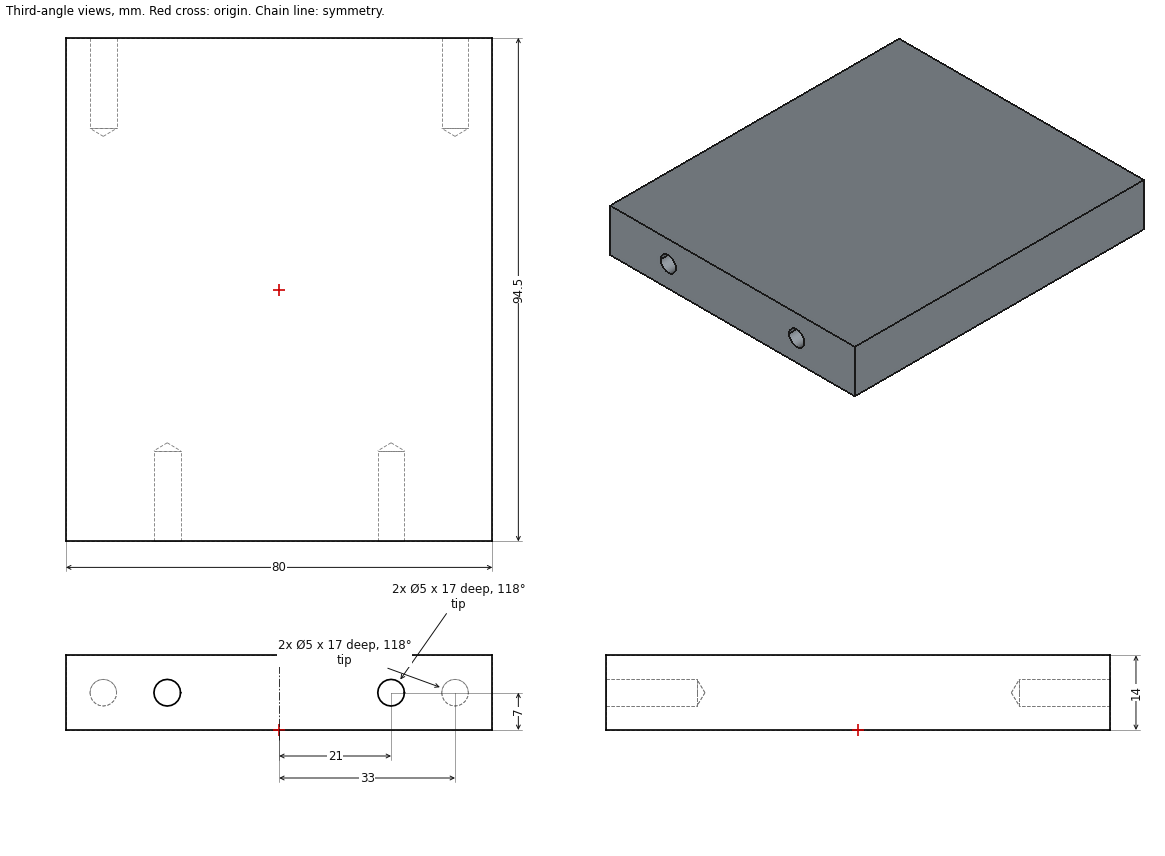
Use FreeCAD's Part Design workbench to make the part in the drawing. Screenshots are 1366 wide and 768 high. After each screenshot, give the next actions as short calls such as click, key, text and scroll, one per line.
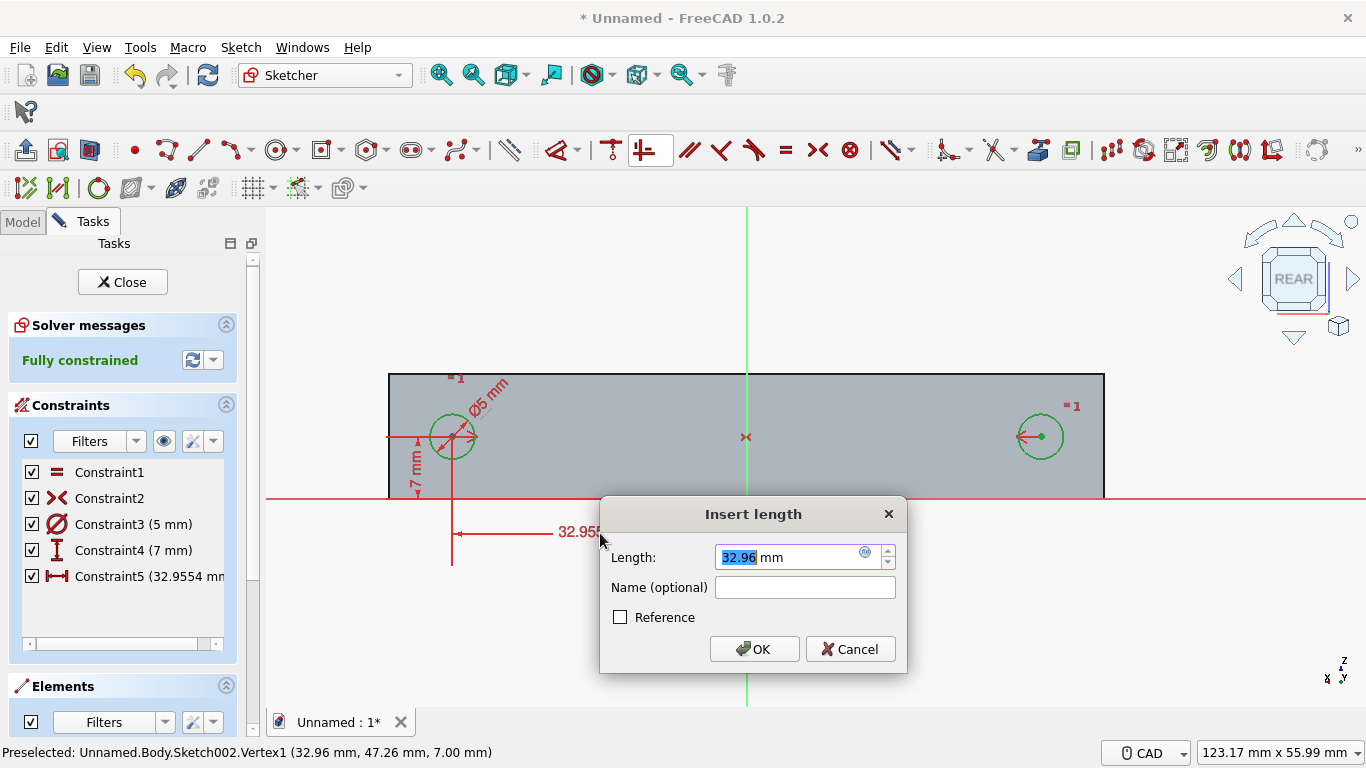
text(33)
key(Return)
key(Escape)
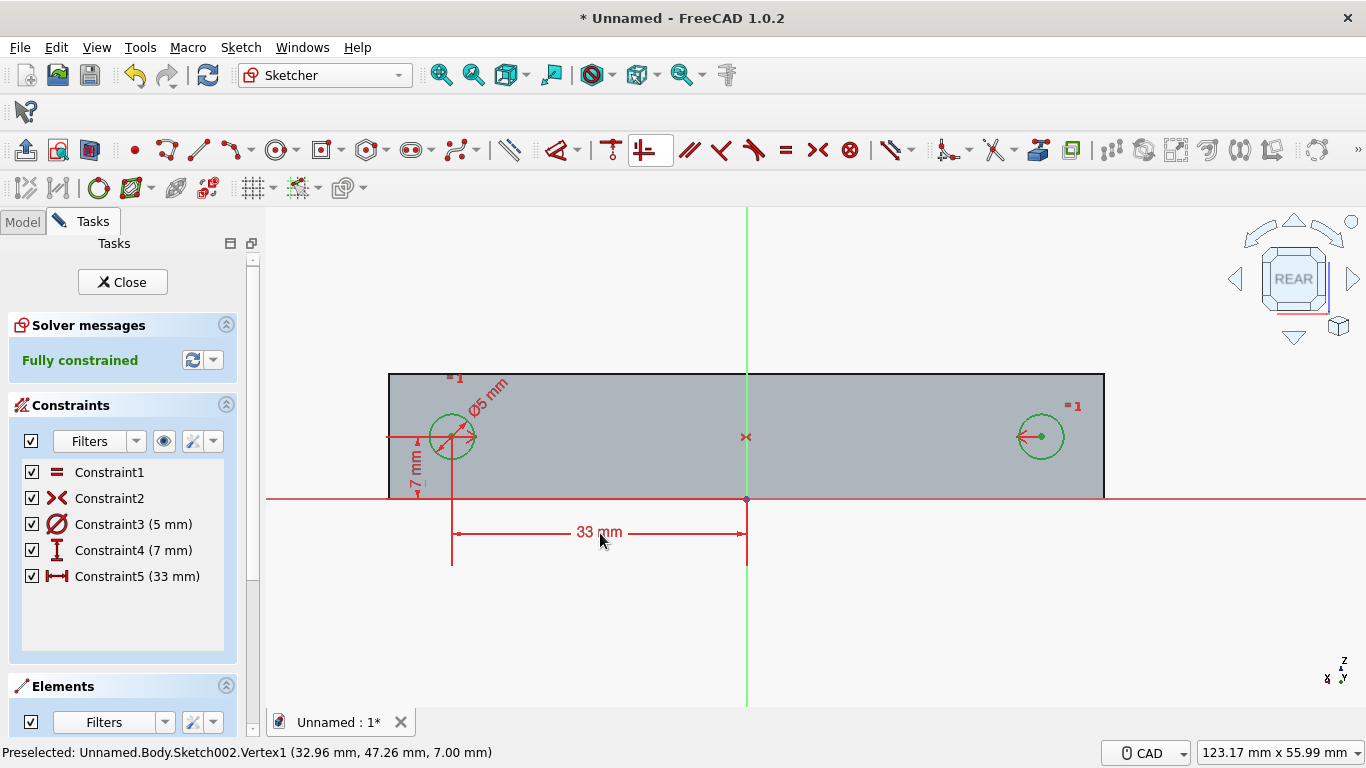
click(123, 282)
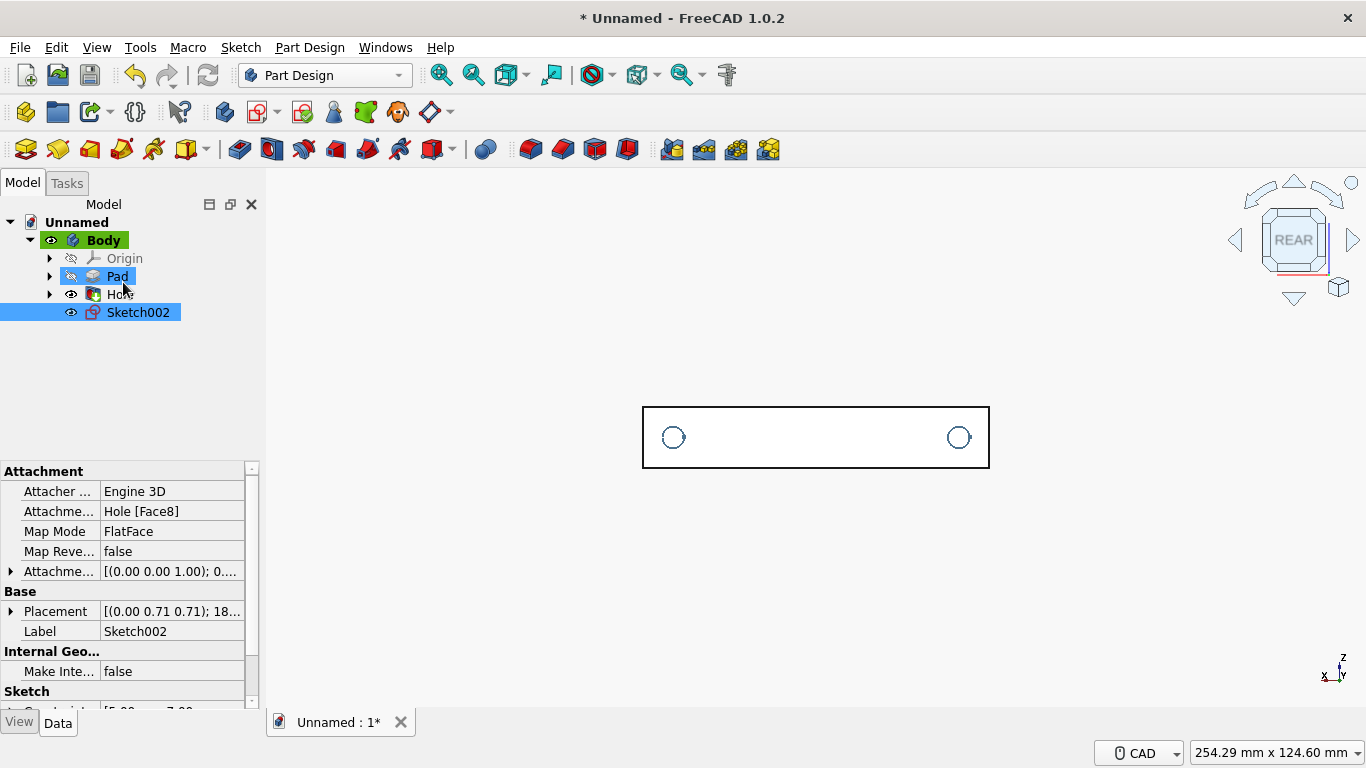
click(272, 150)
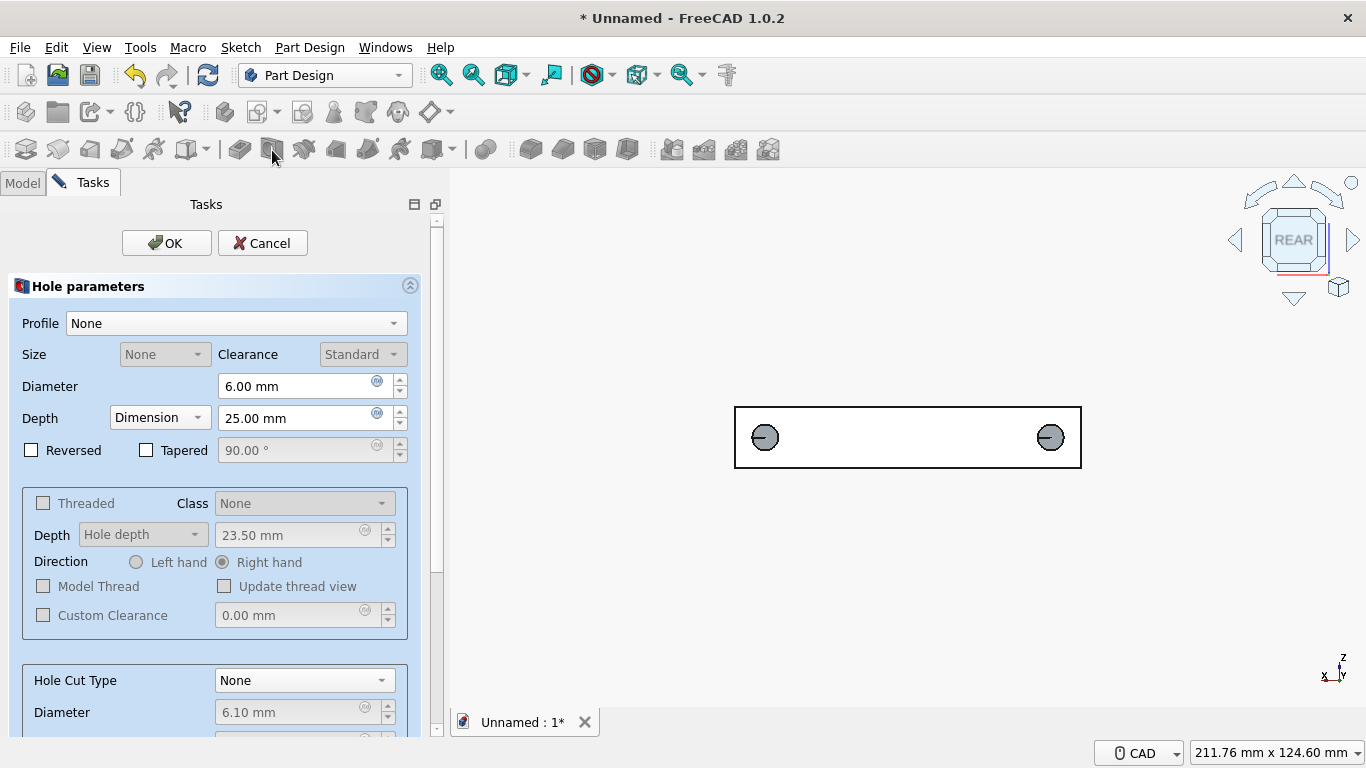
triple_click(305, 386)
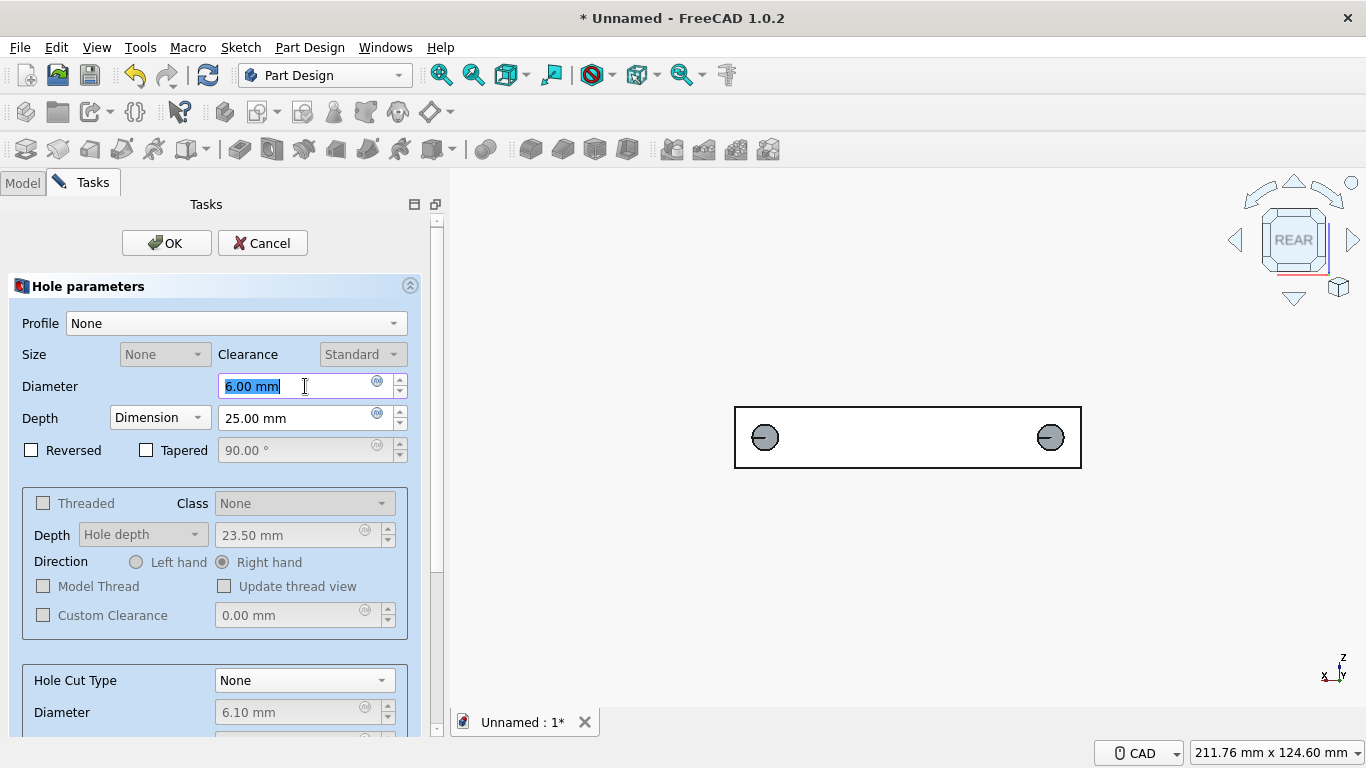
text(5)
key(Tab)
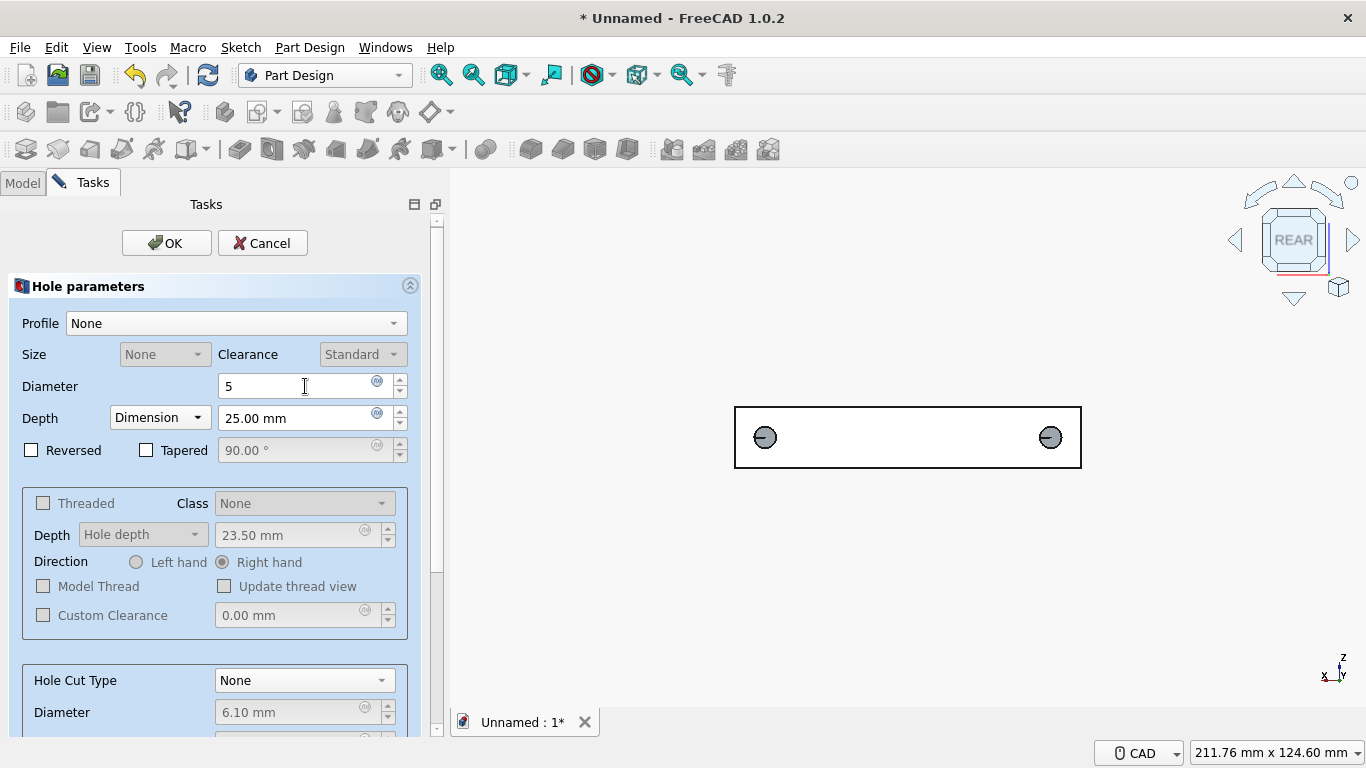
triple_click(305, 418)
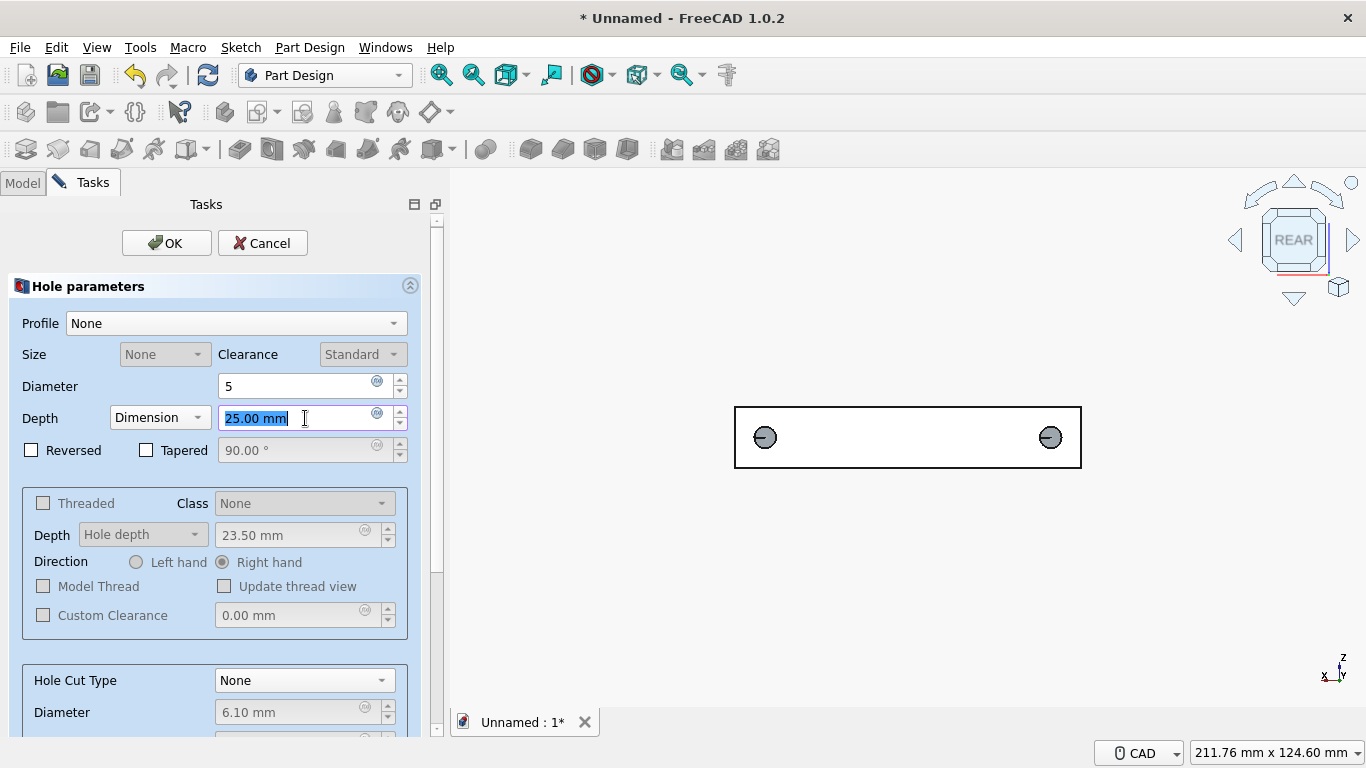
text(17)
key(Tab)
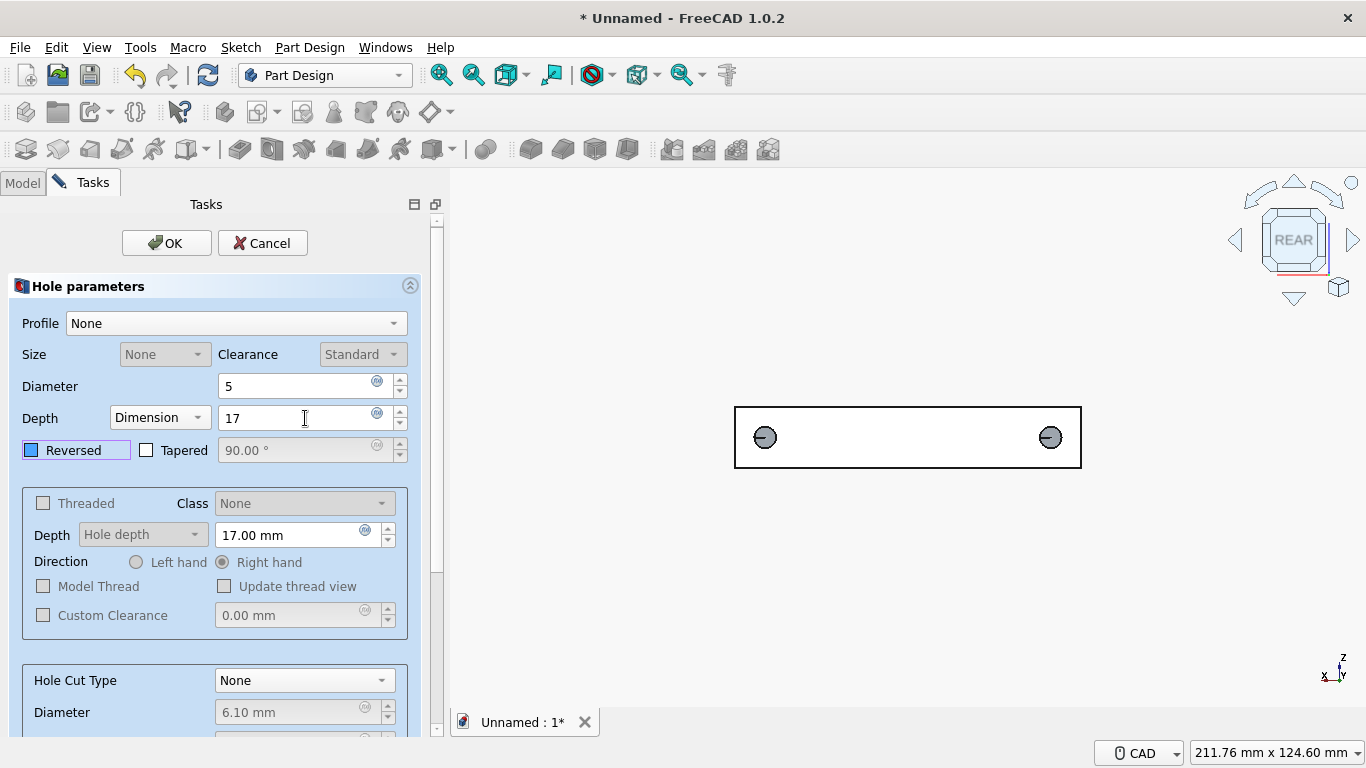
click(167, 243)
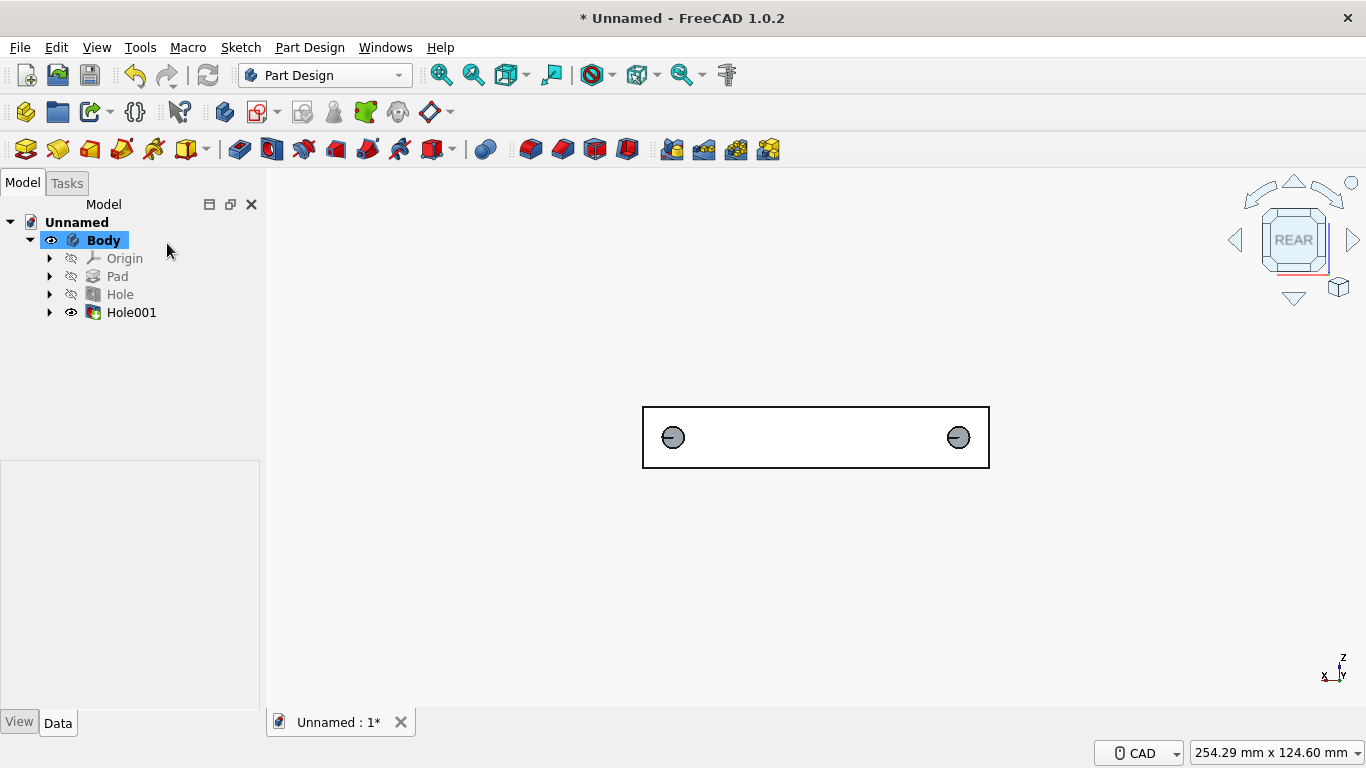
key(0)